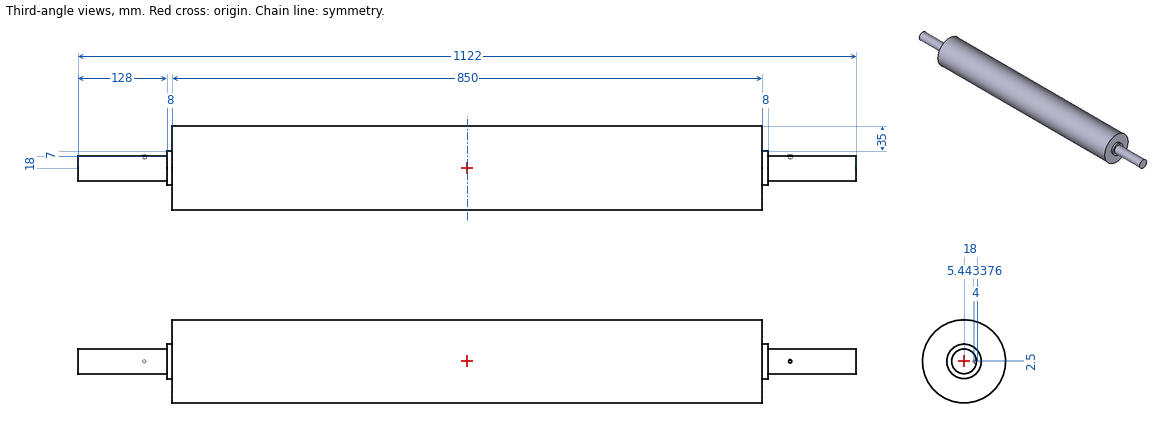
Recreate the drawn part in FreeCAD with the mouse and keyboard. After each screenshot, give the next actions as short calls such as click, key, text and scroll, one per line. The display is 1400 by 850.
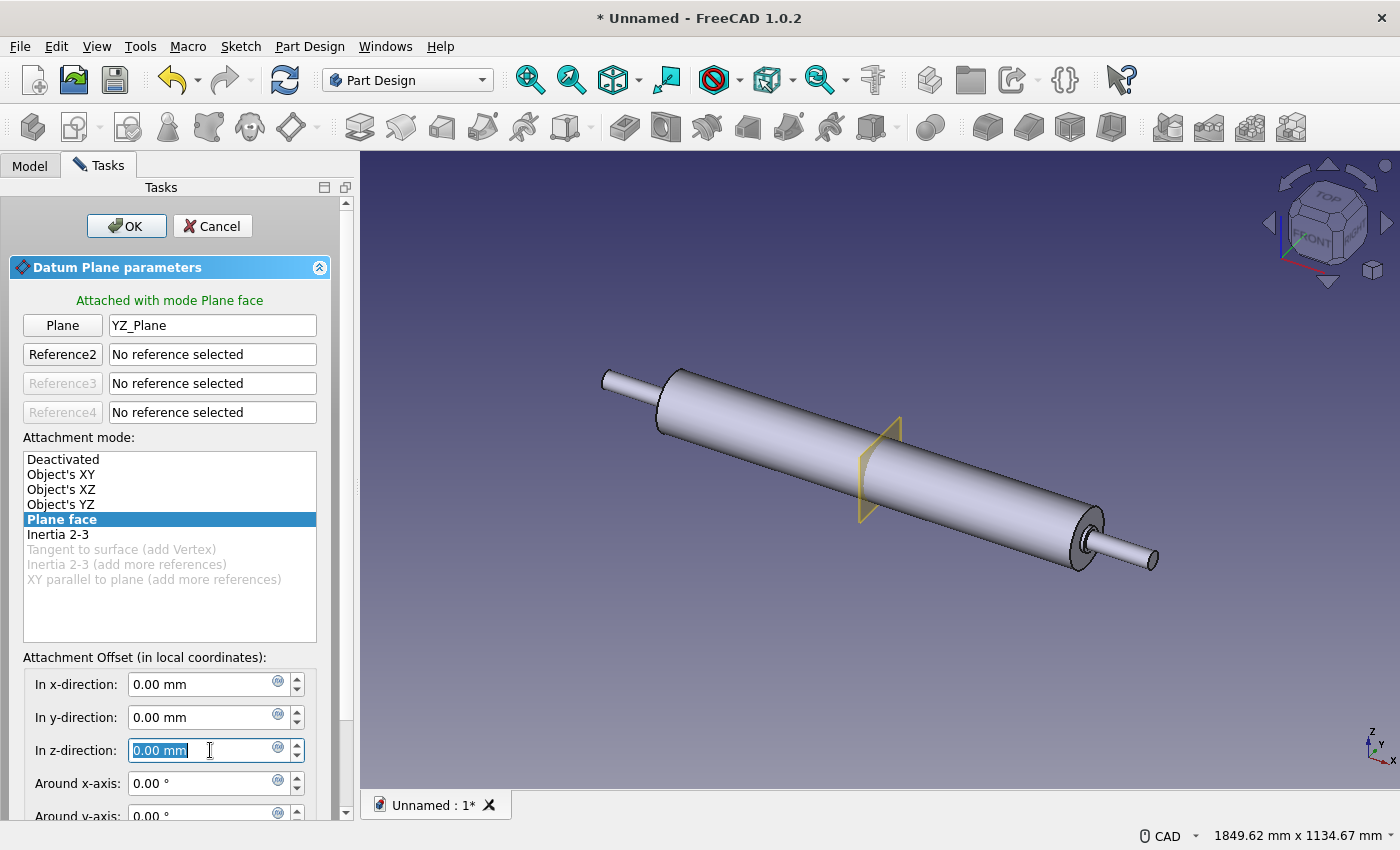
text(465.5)
key(Tab)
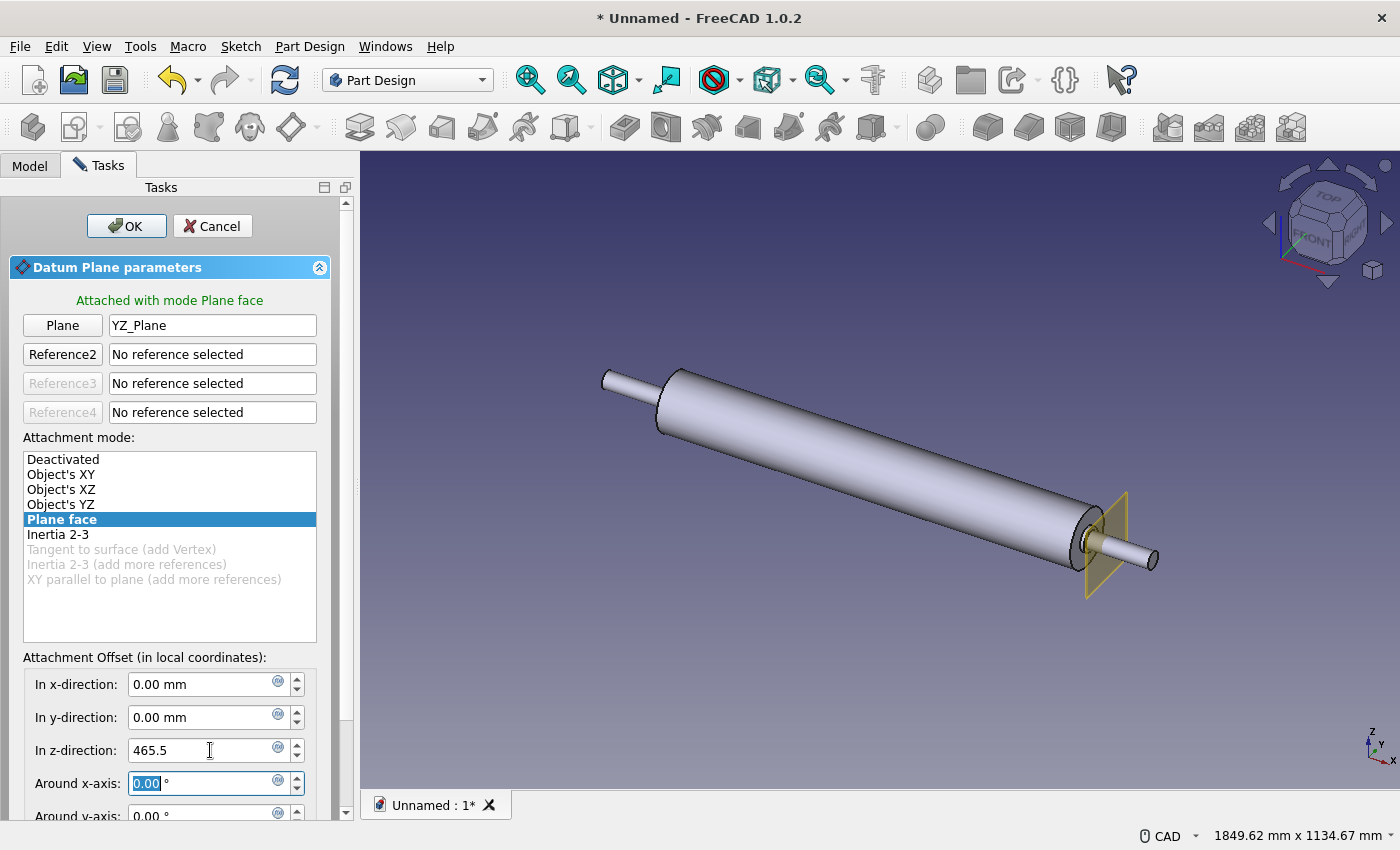
click(127, 226)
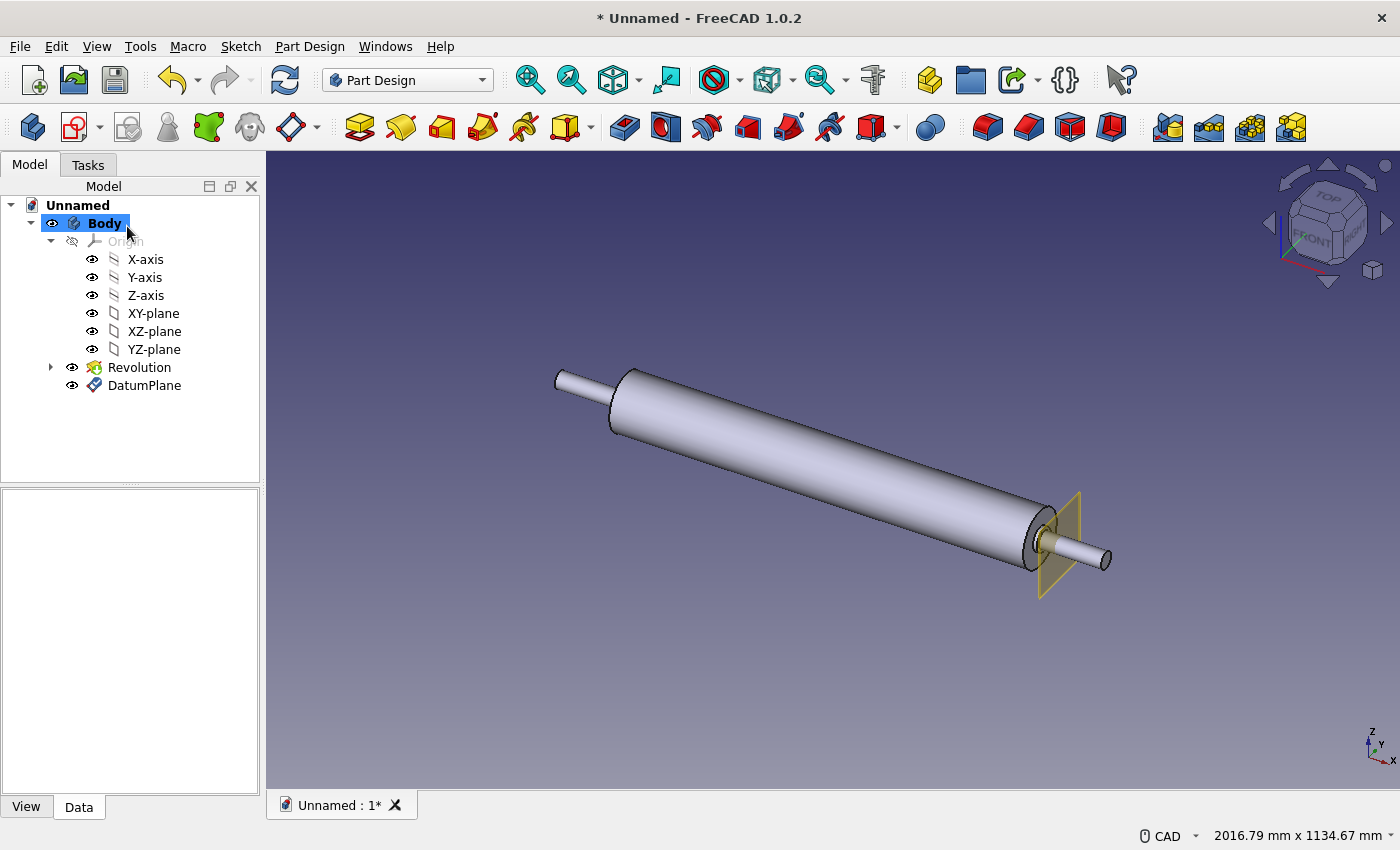
click(117, 385)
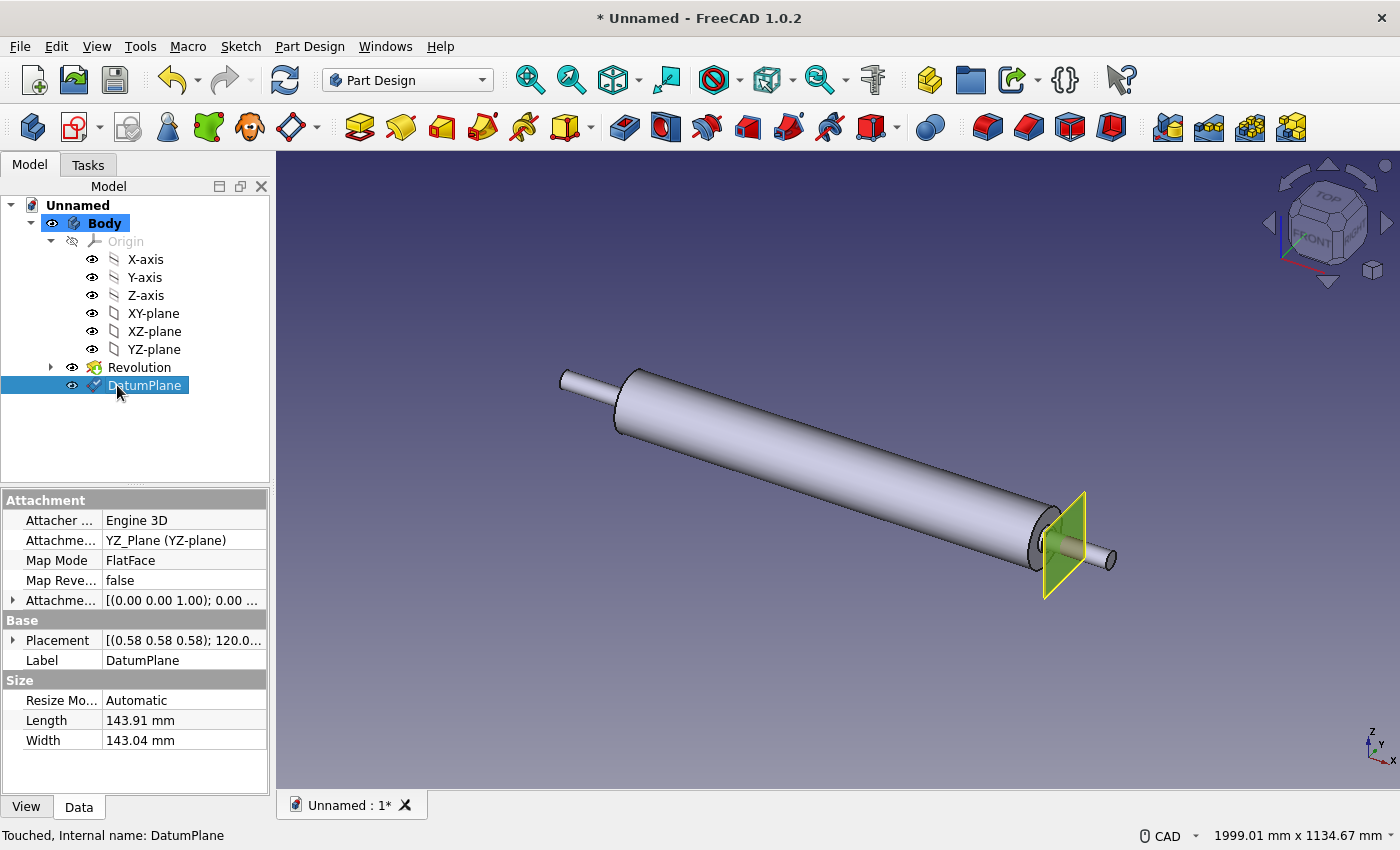
click(74, 128)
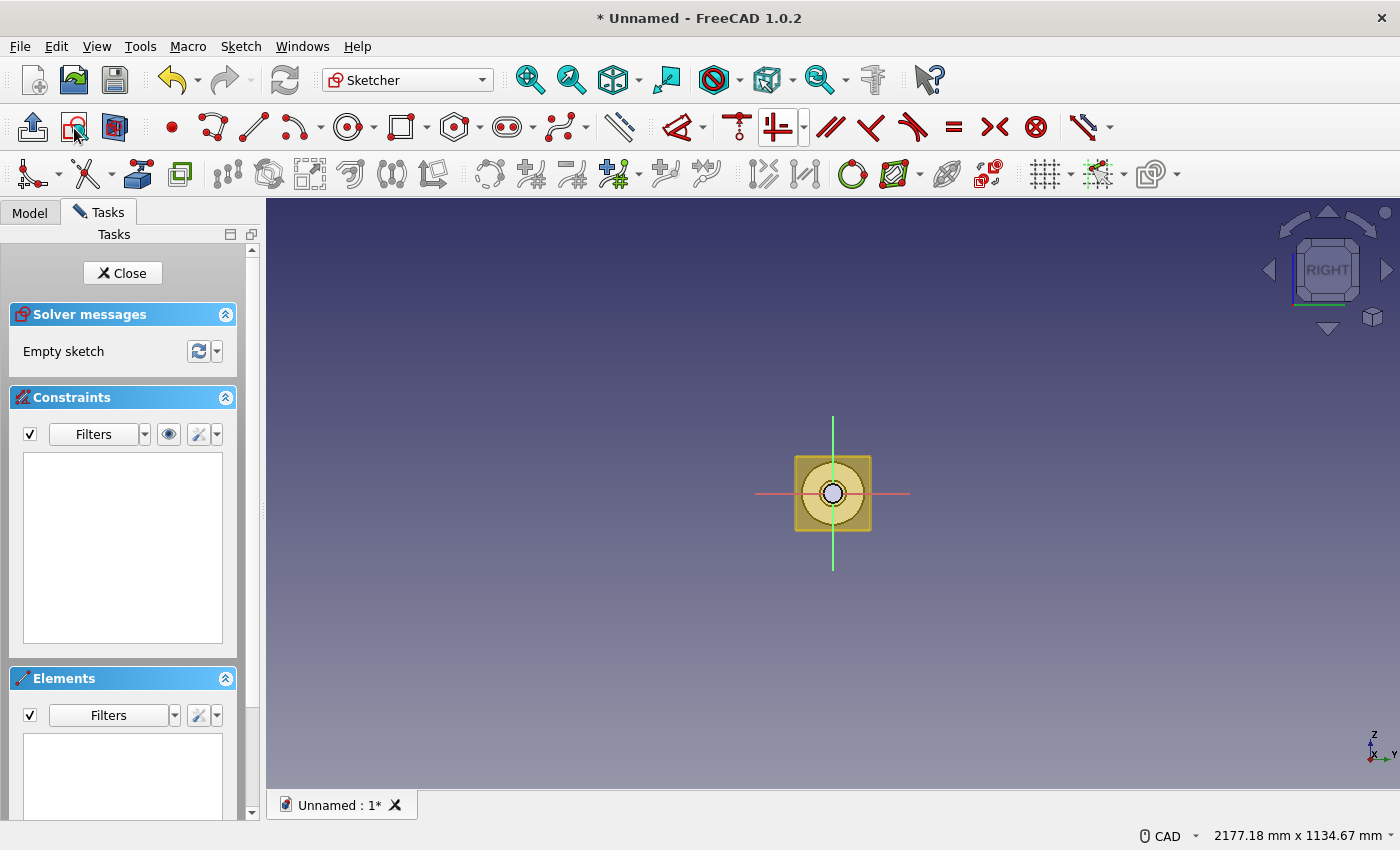
key(q)
key(s)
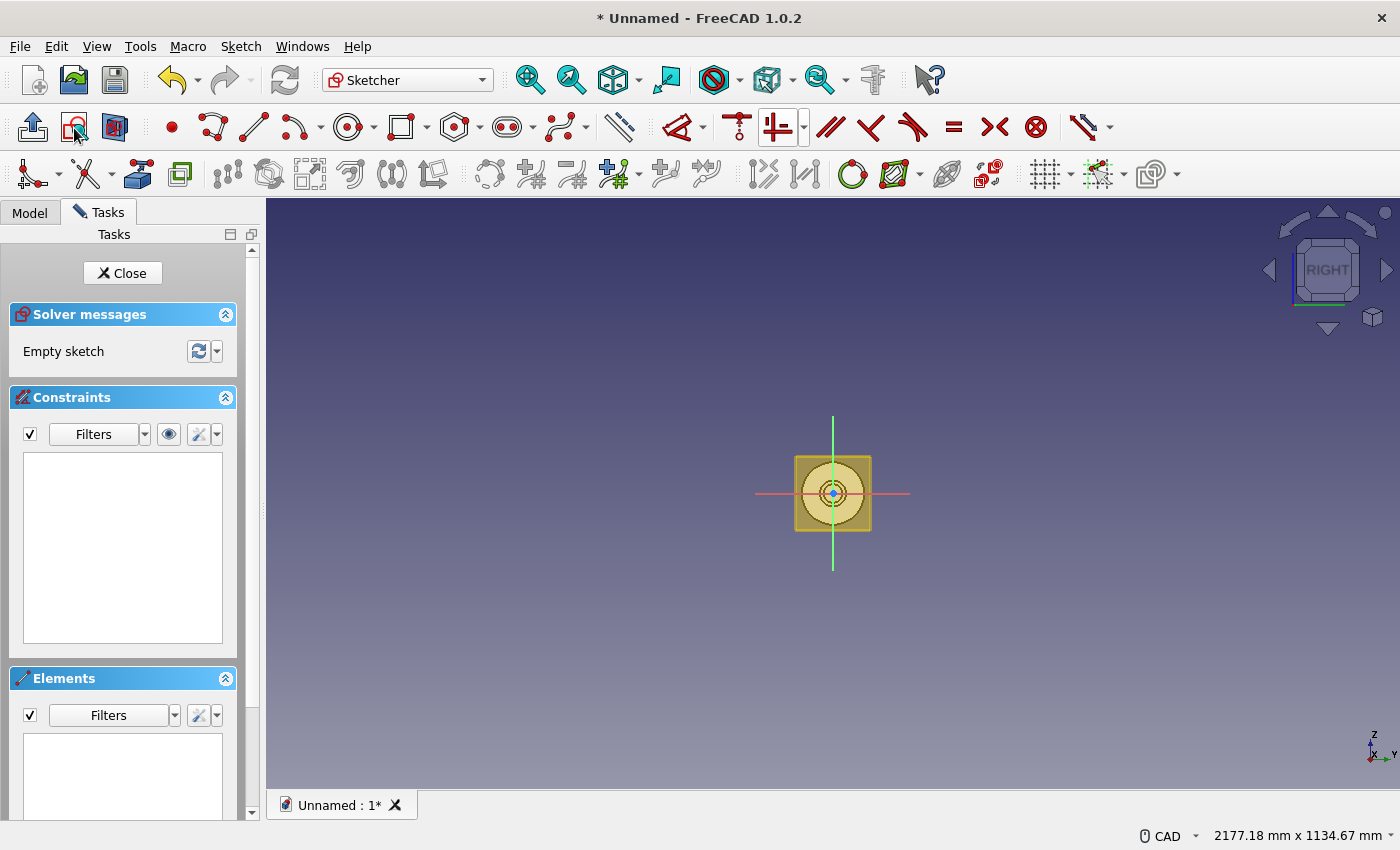
scroll(845, 493, up, 15)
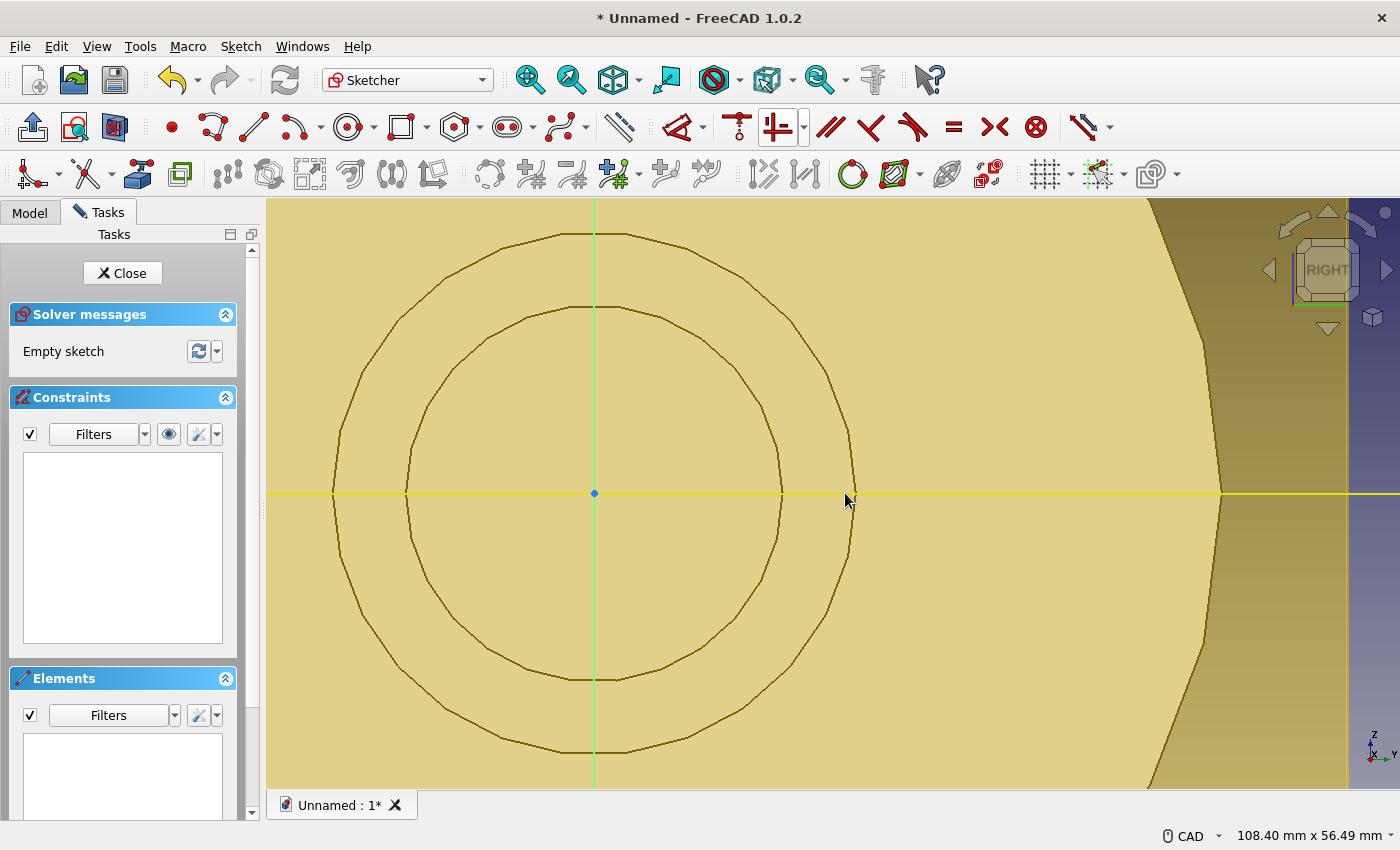
scroll(753, 479, up, 12)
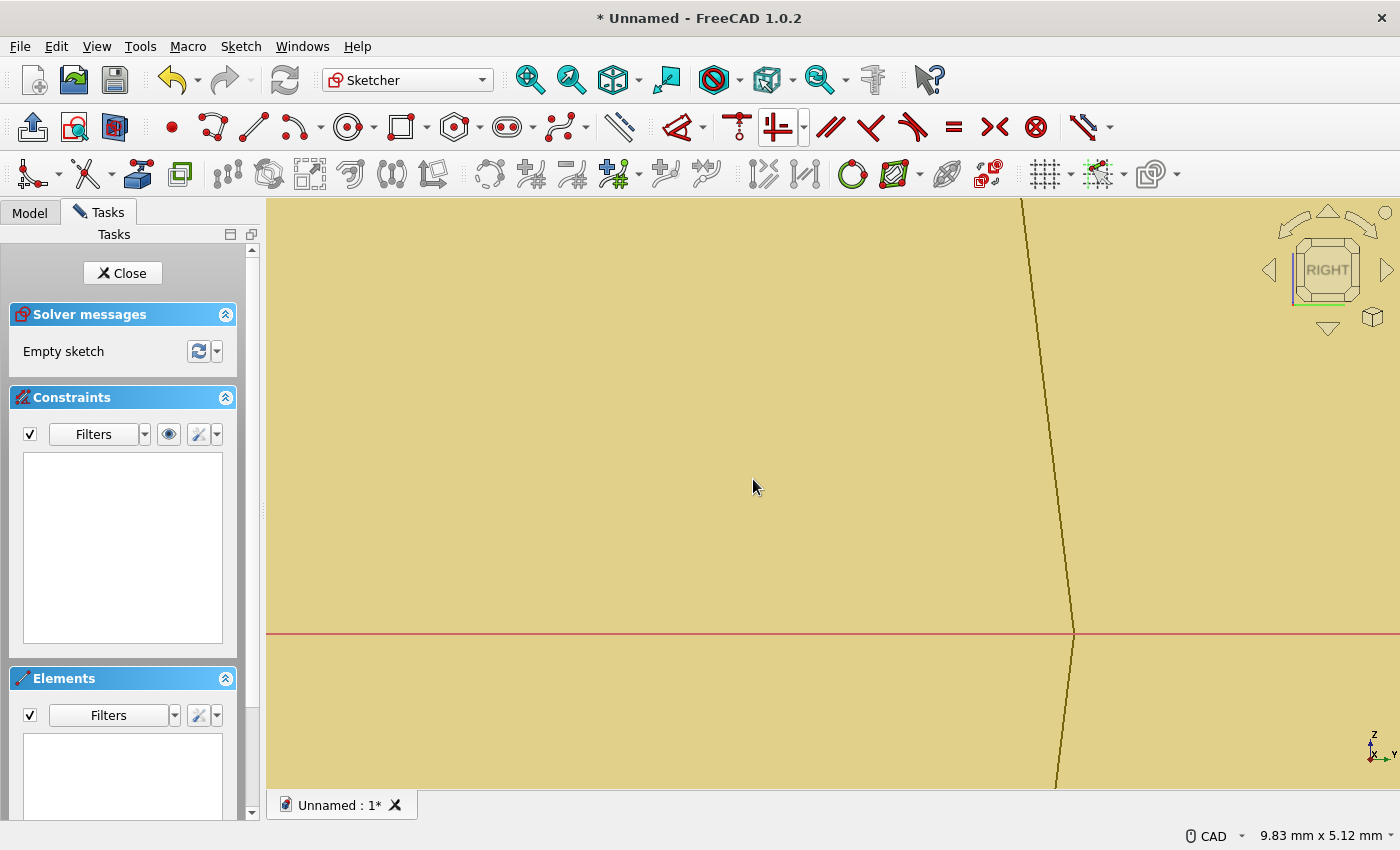
click(213, 128)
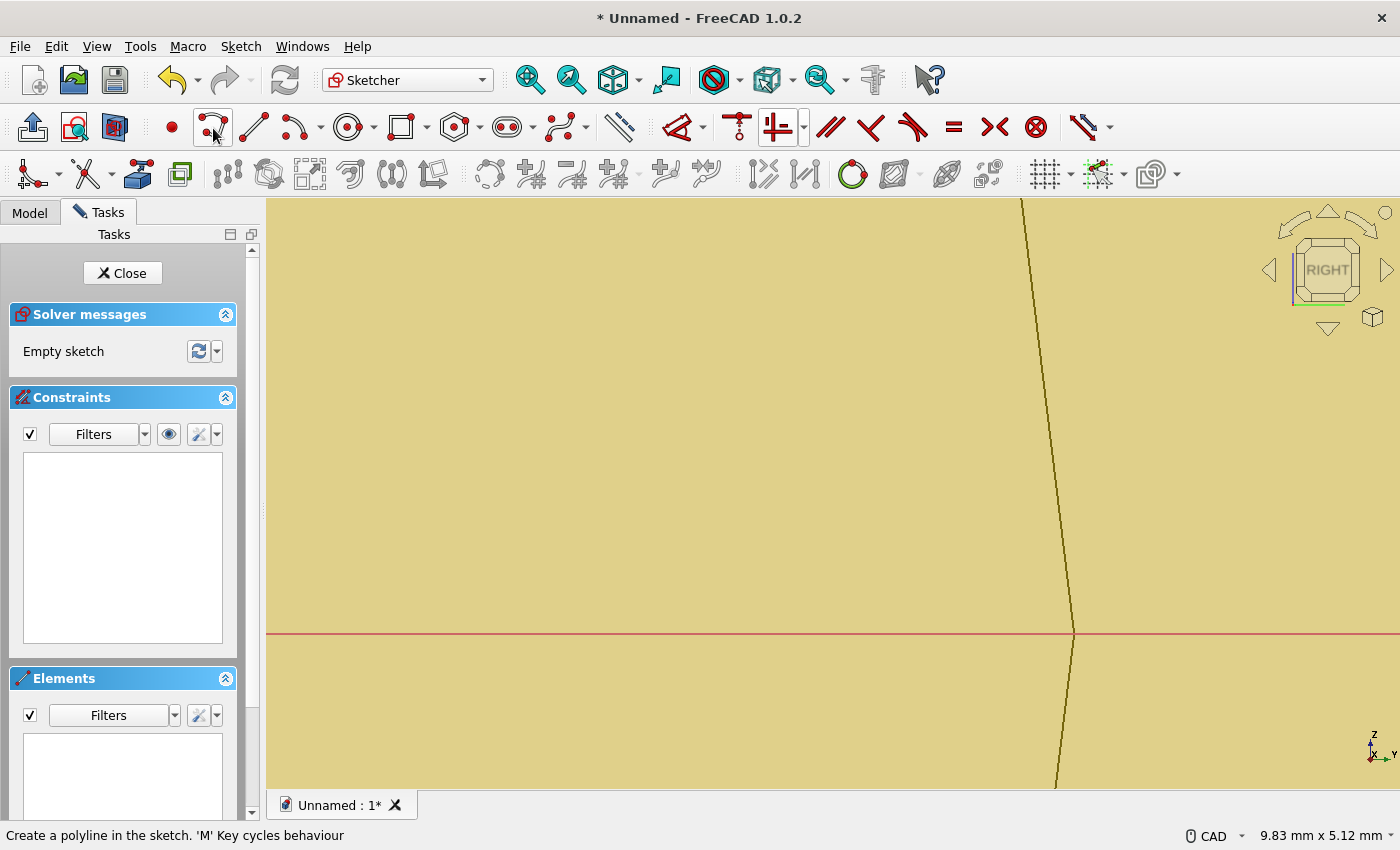
click(446, 634)
click(1074, 625)
click(1074, 346)
click(613, 346)
click(446, 634)
key(Escape)
key(Escape)